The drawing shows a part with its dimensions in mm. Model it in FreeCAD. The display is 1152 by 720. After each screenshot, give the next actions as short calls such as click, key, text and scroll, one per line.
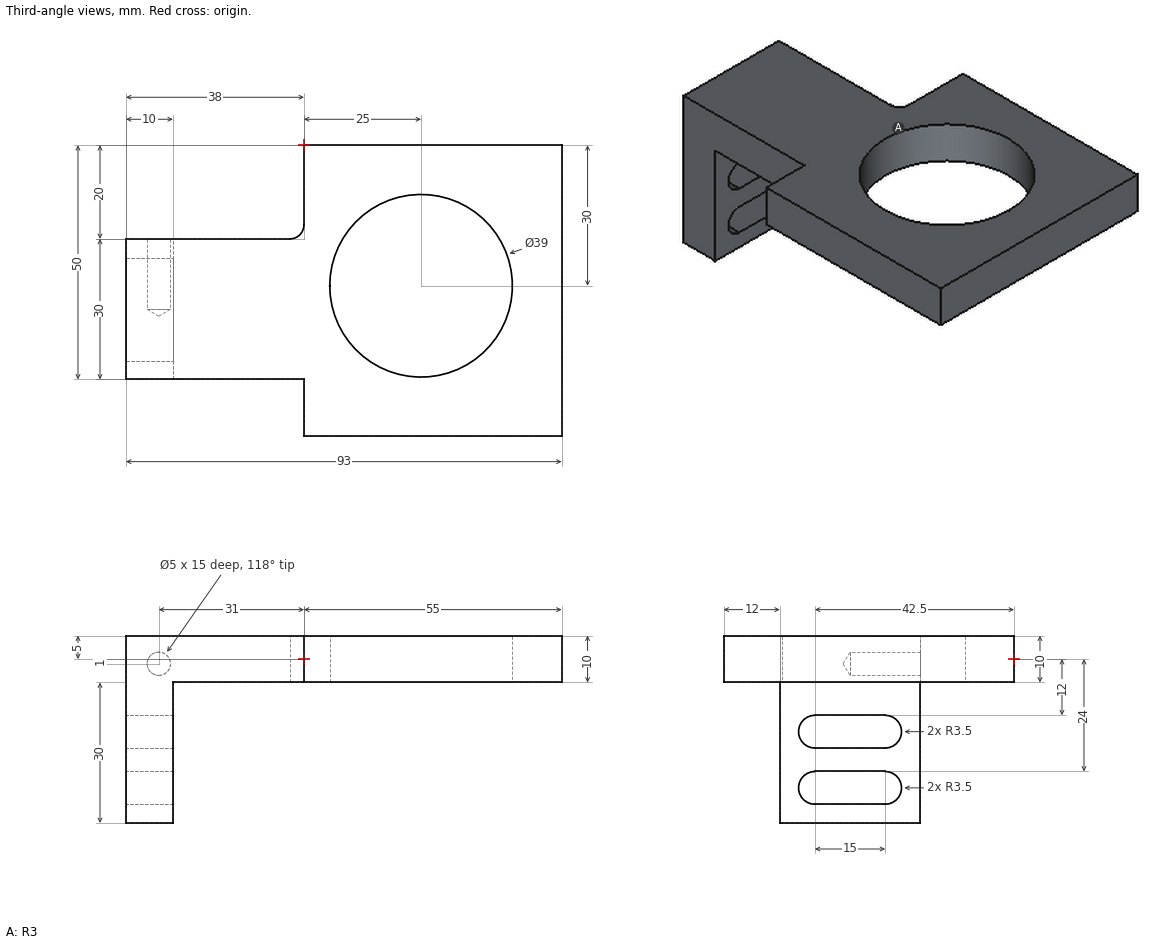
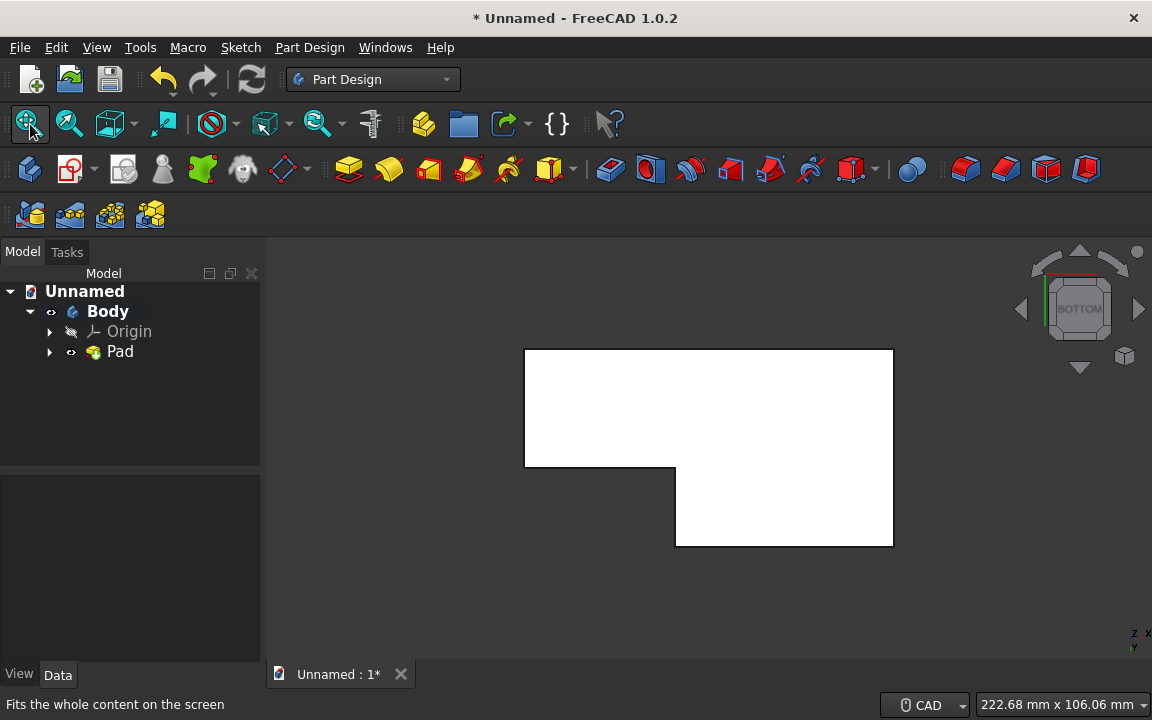
key(4)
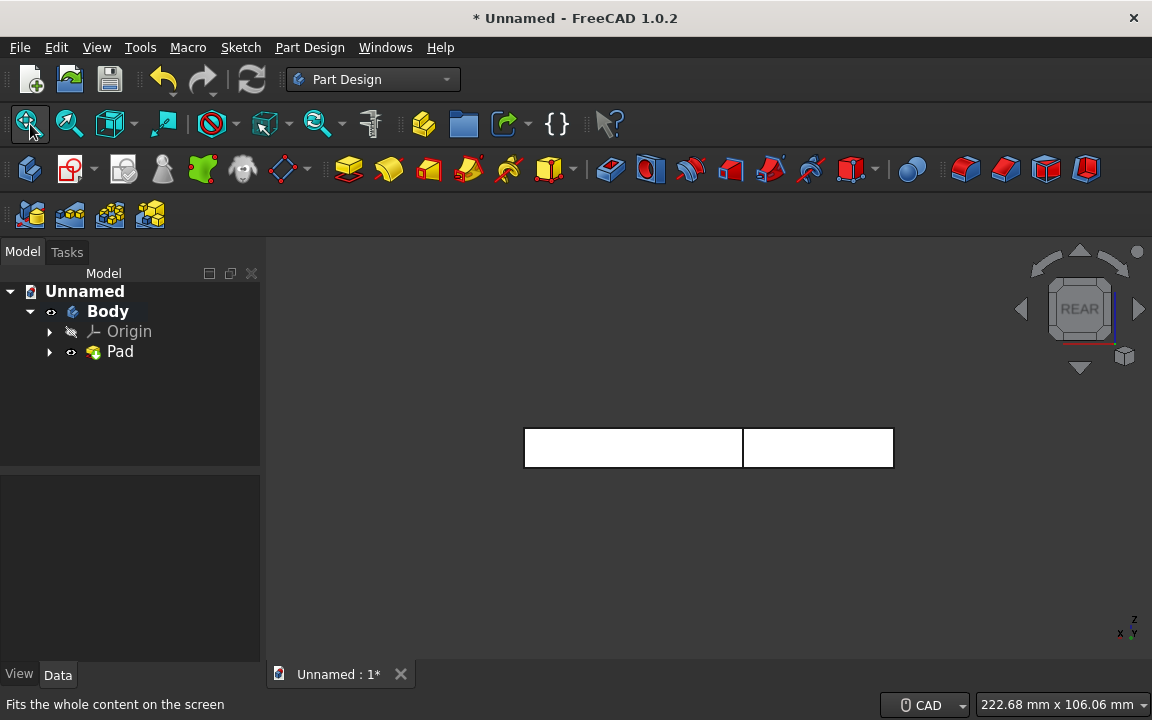
click(30, 124)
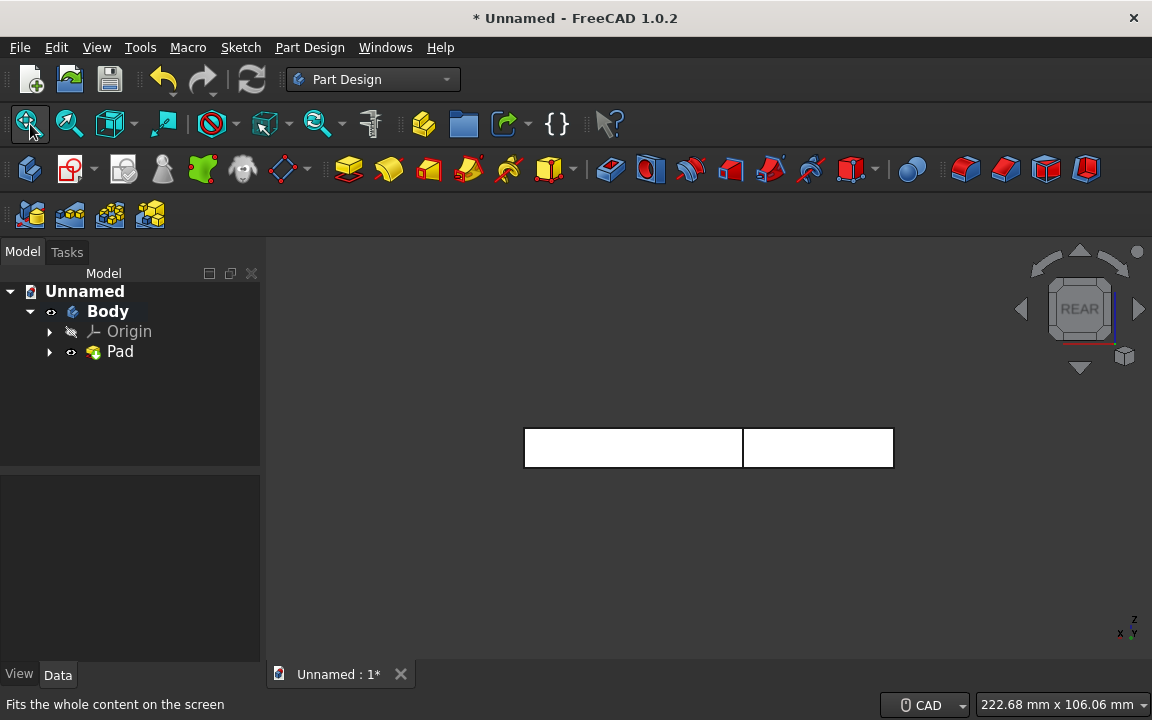
key(6)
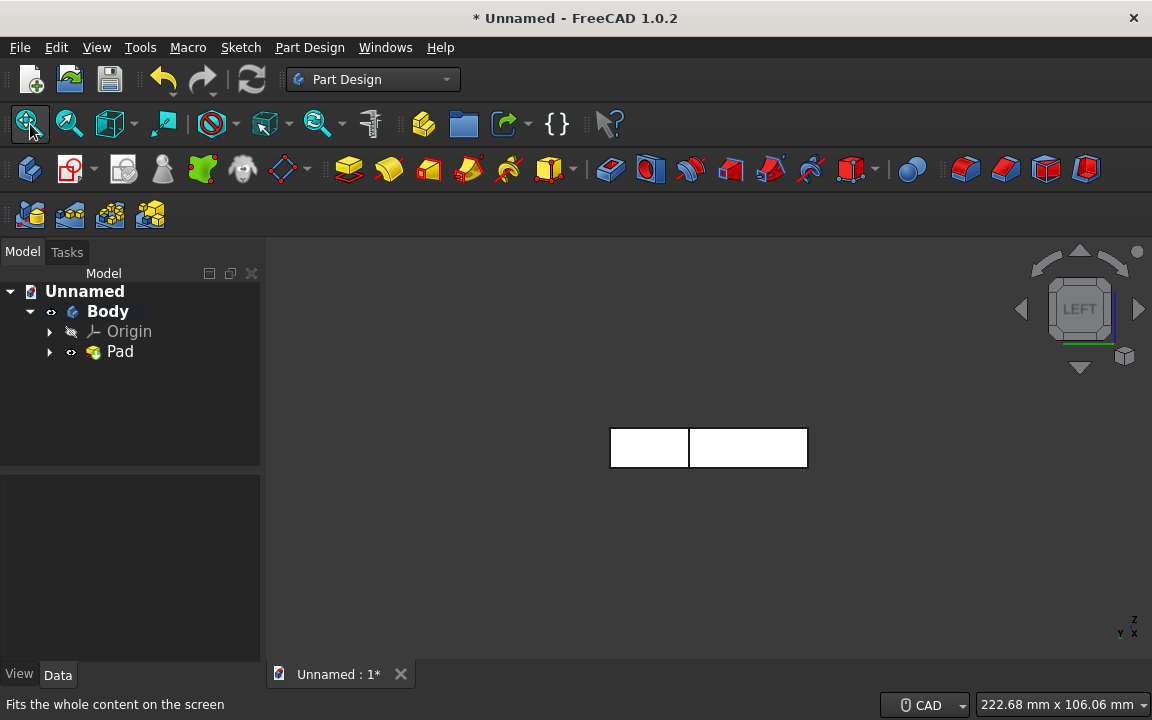
key(v)
key(f)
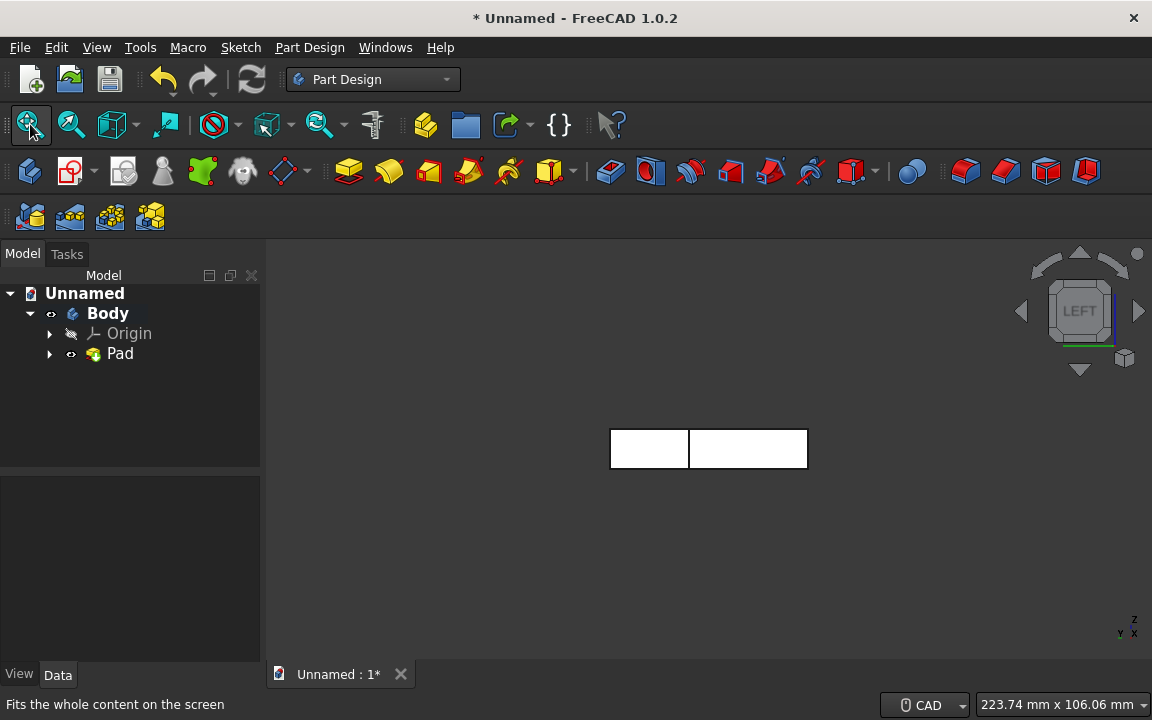
key(v)
key(3)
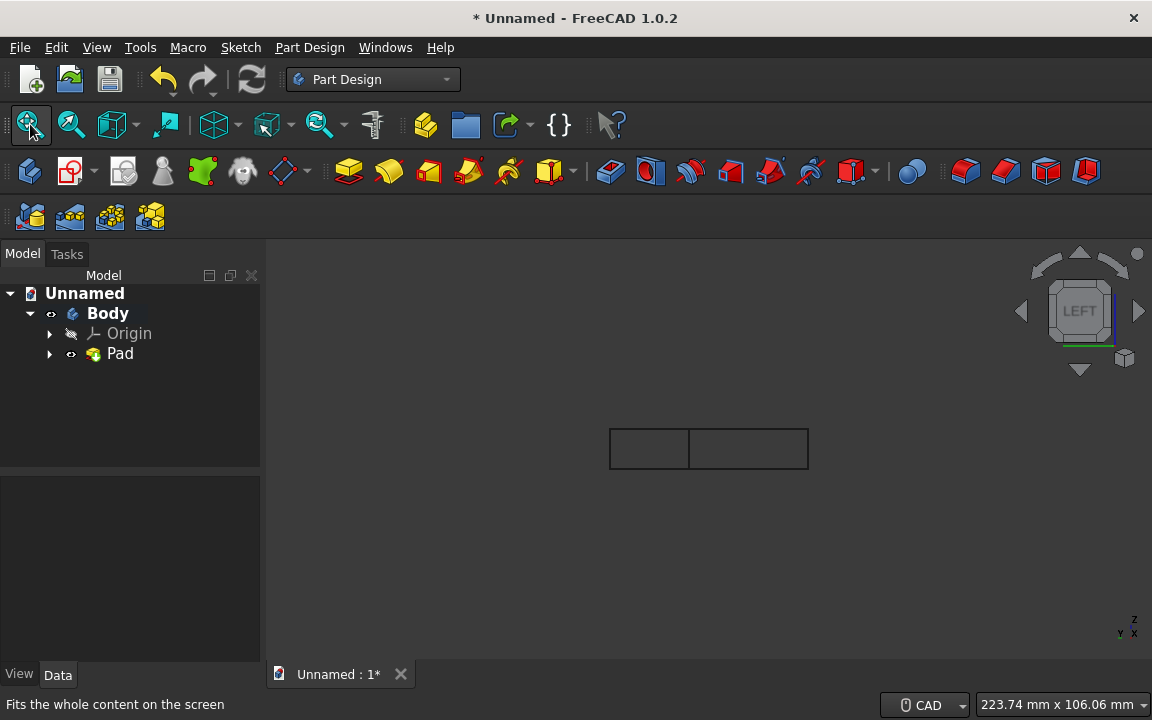
key(0)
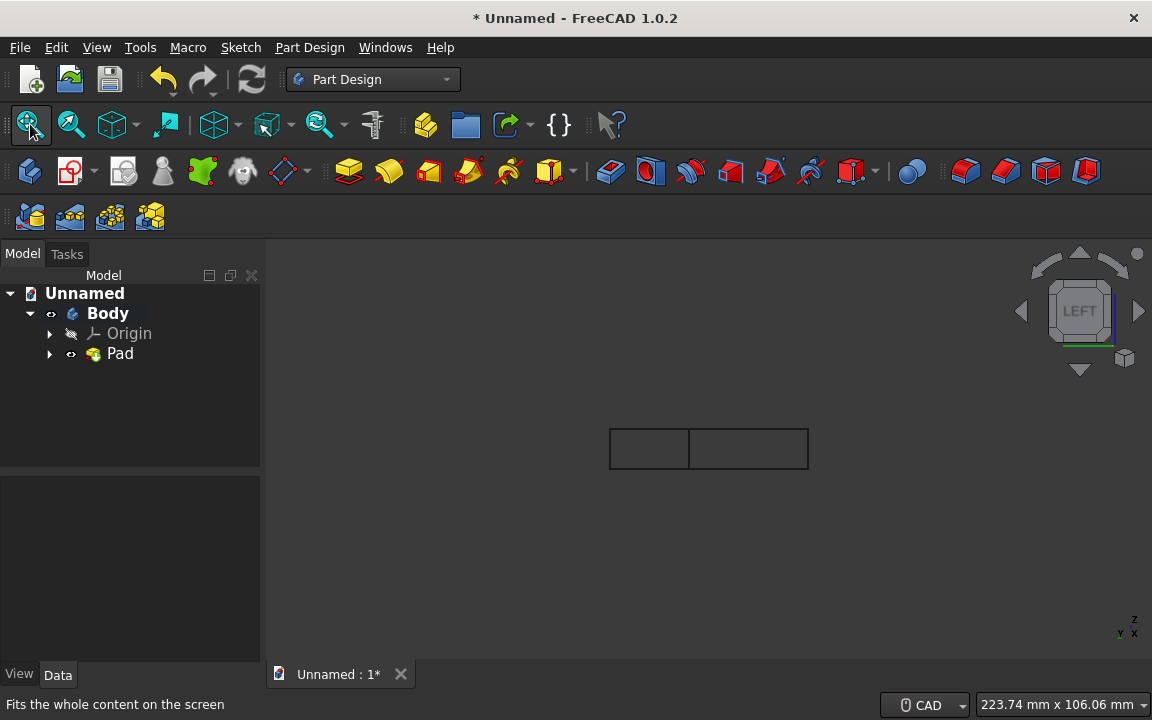
click(699, 426)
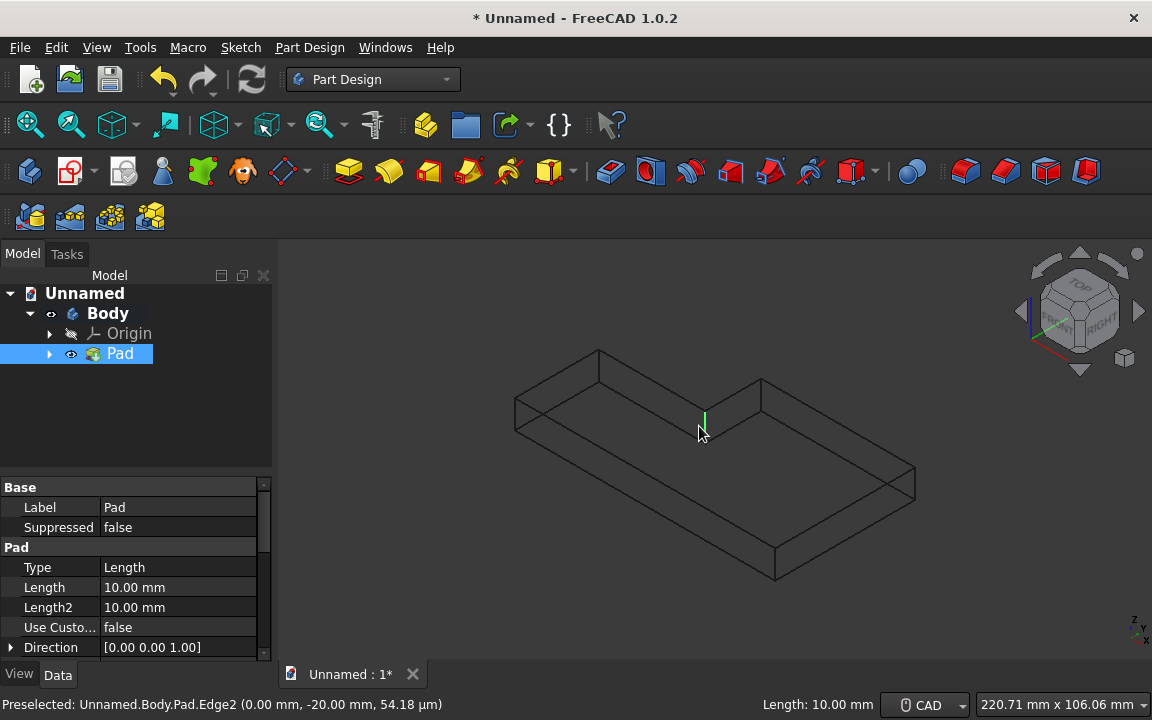
key(v)
key(1)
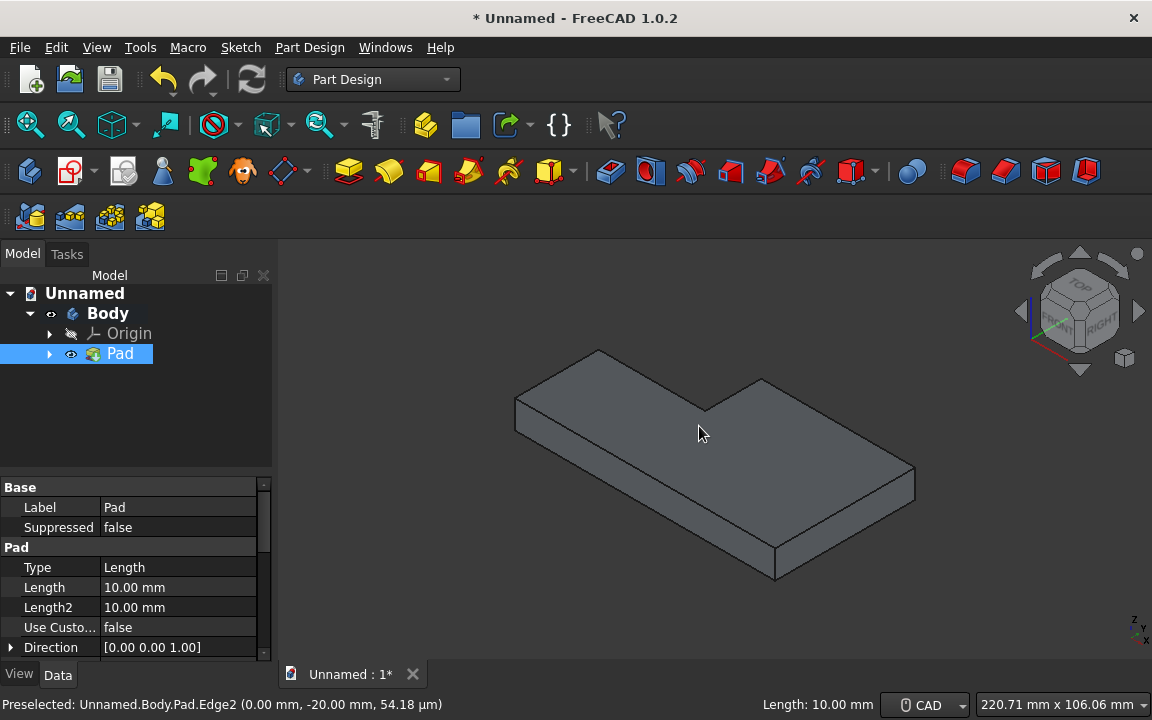
click(966, 172)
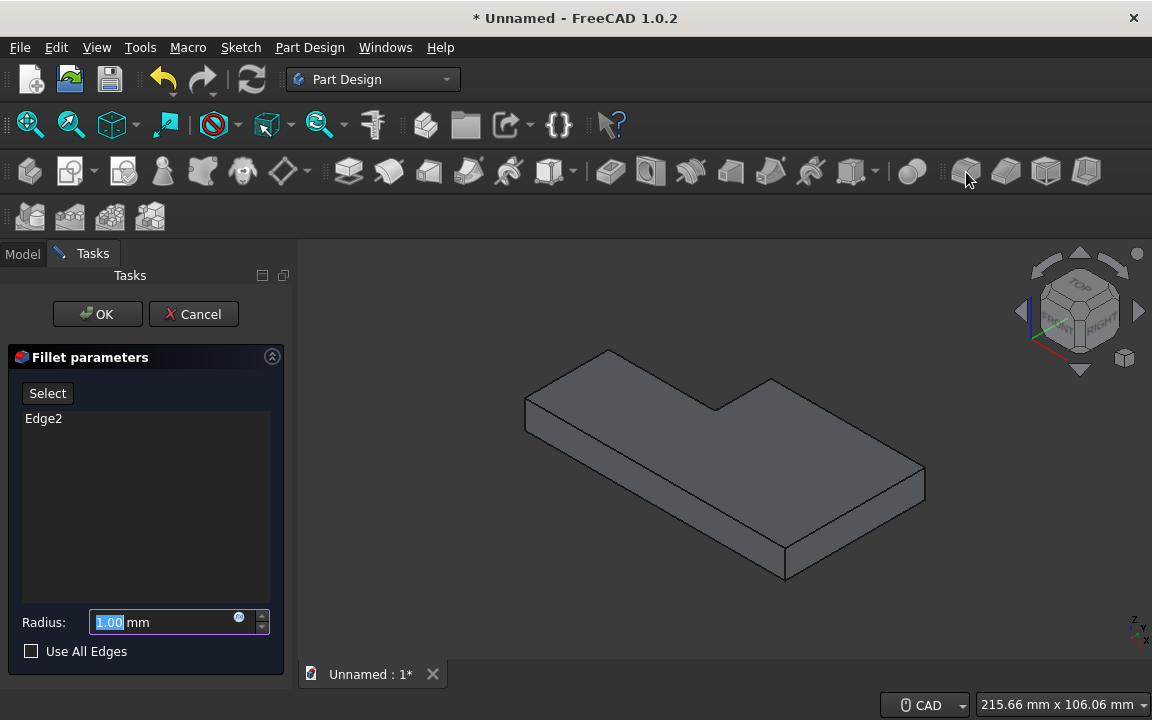
text(3)
key(Tab)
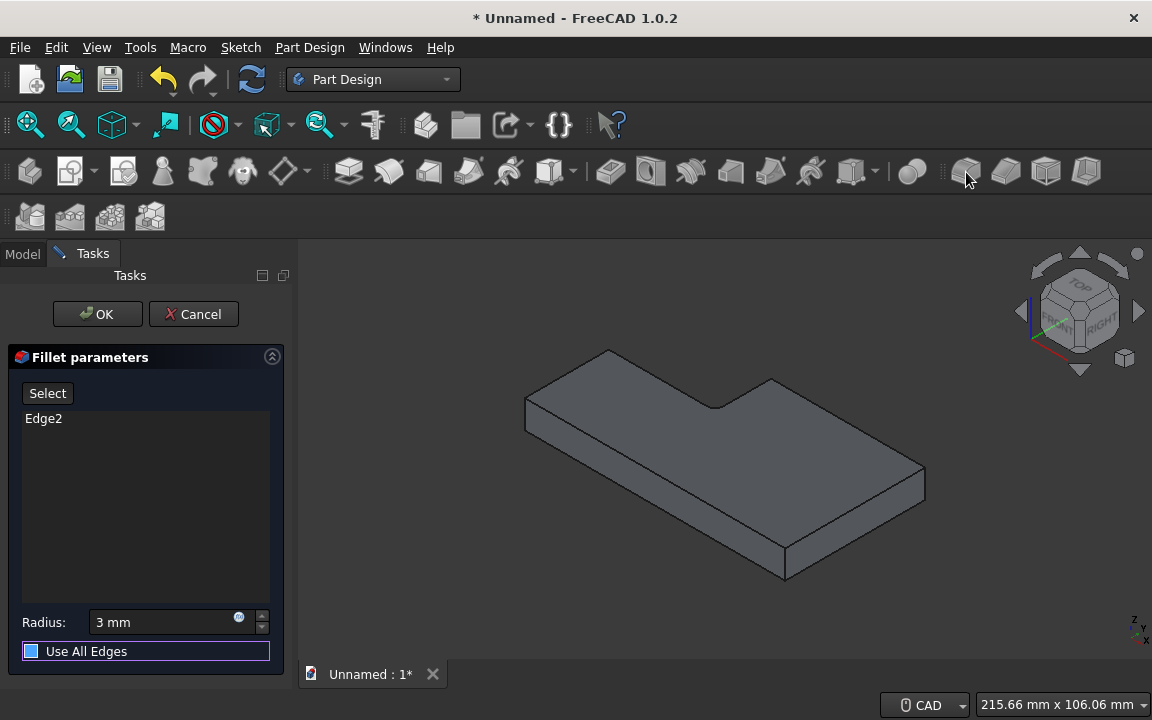
click(98, 314)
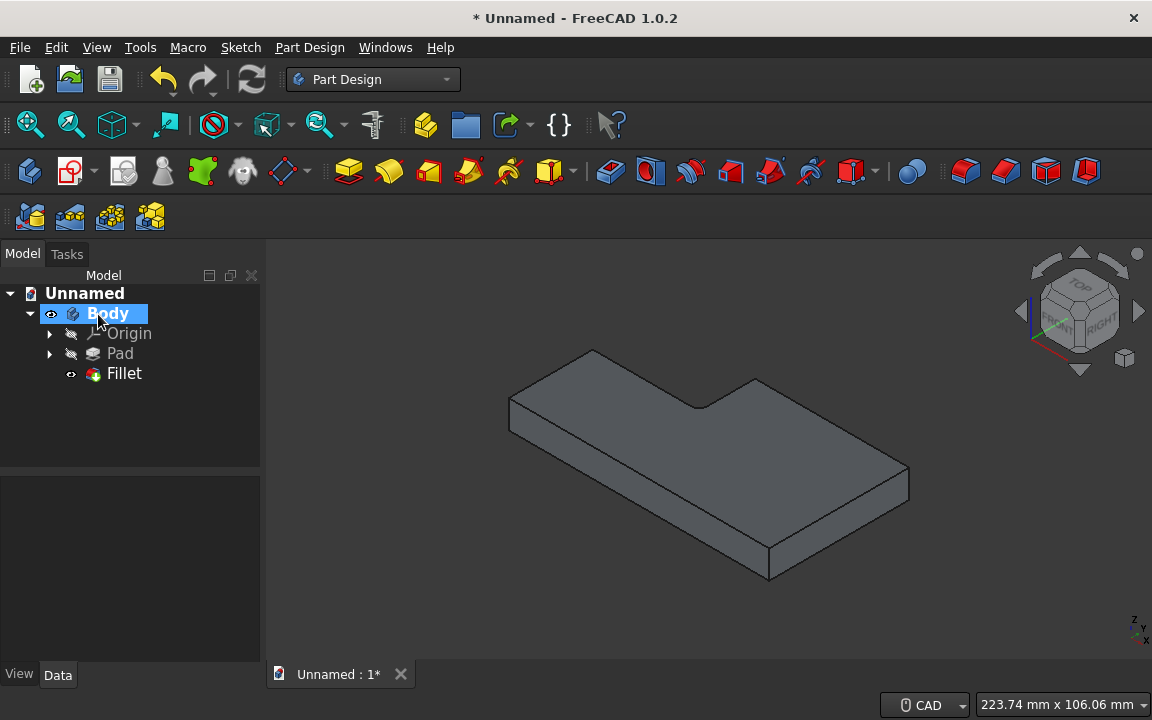
key(5)